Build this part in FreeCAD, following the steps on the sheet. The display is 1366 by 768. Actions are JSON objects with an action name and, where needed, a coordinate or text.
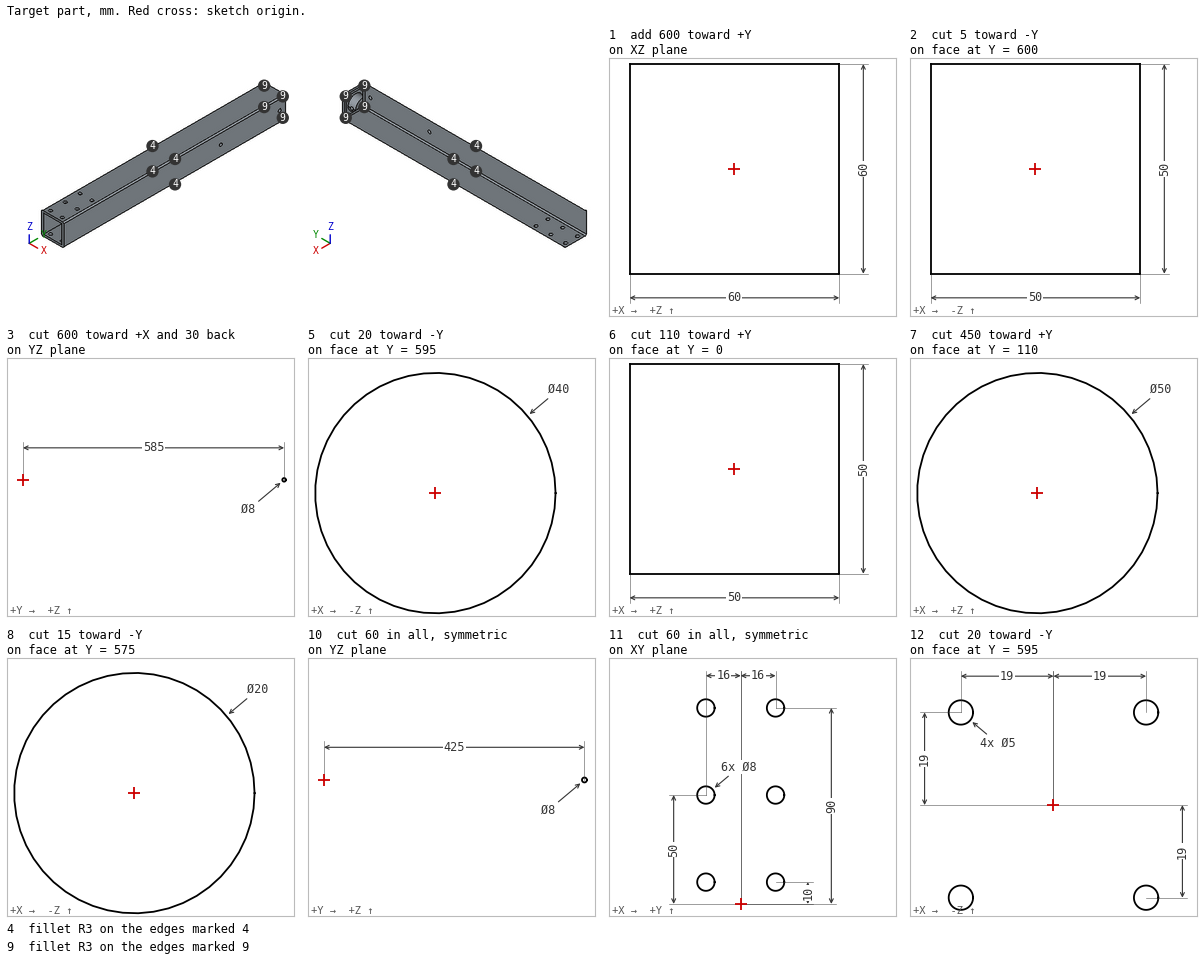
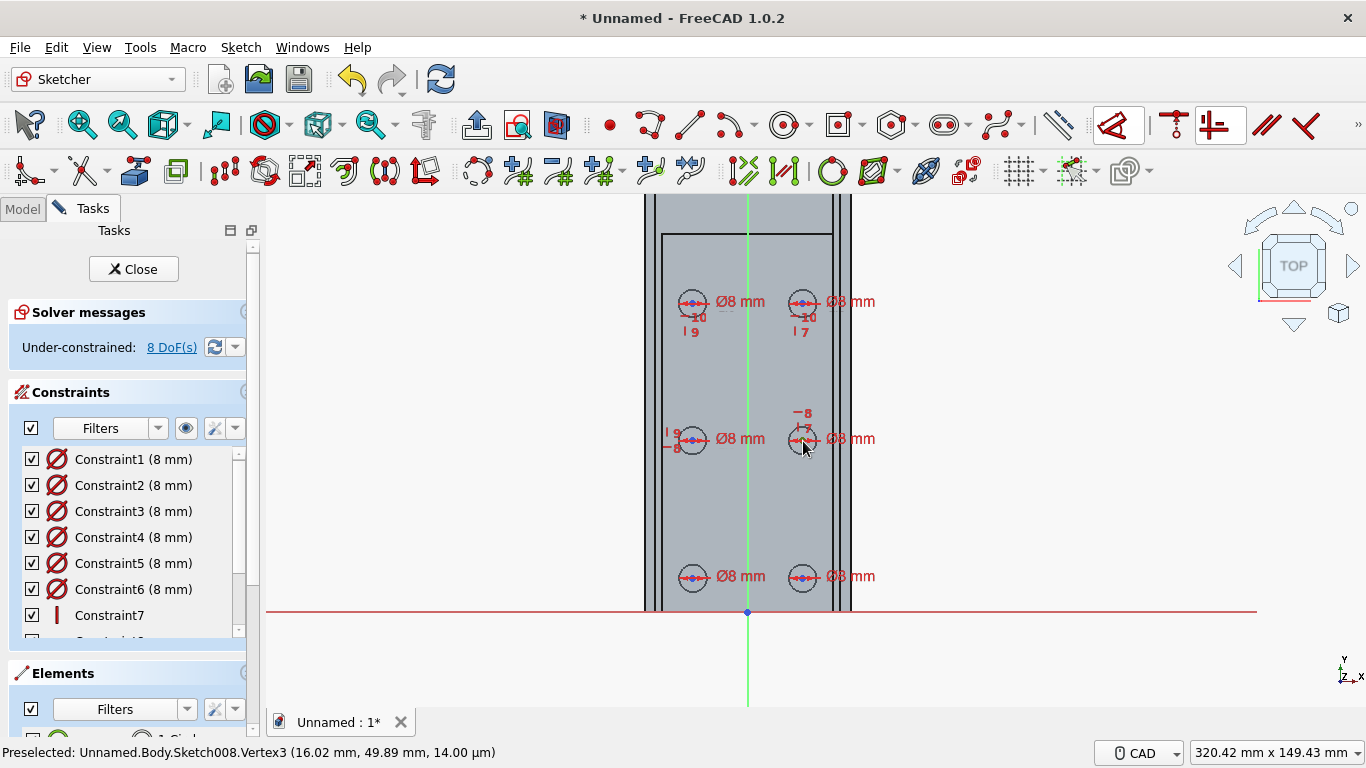
{"action": "left_click", "coordinate": [803, 578]}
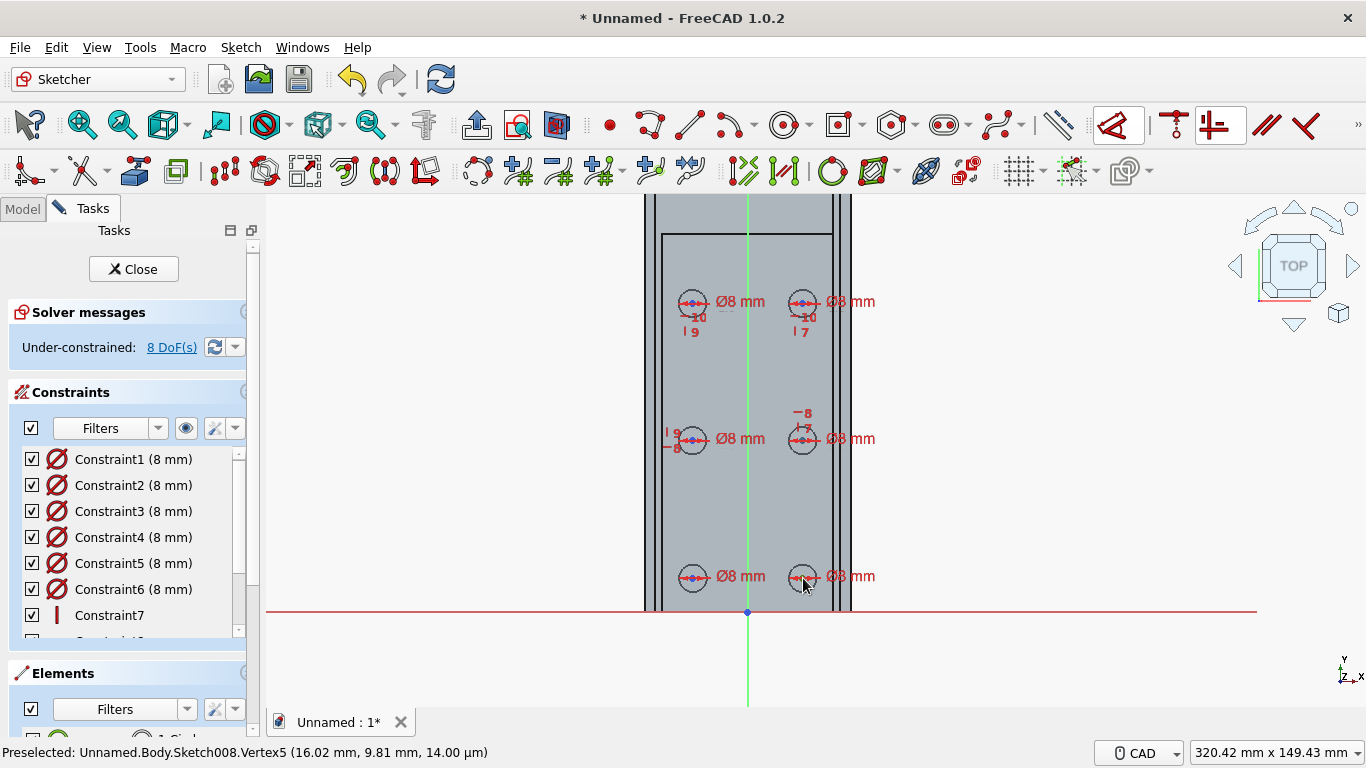
{"action": "key", "text": "v"}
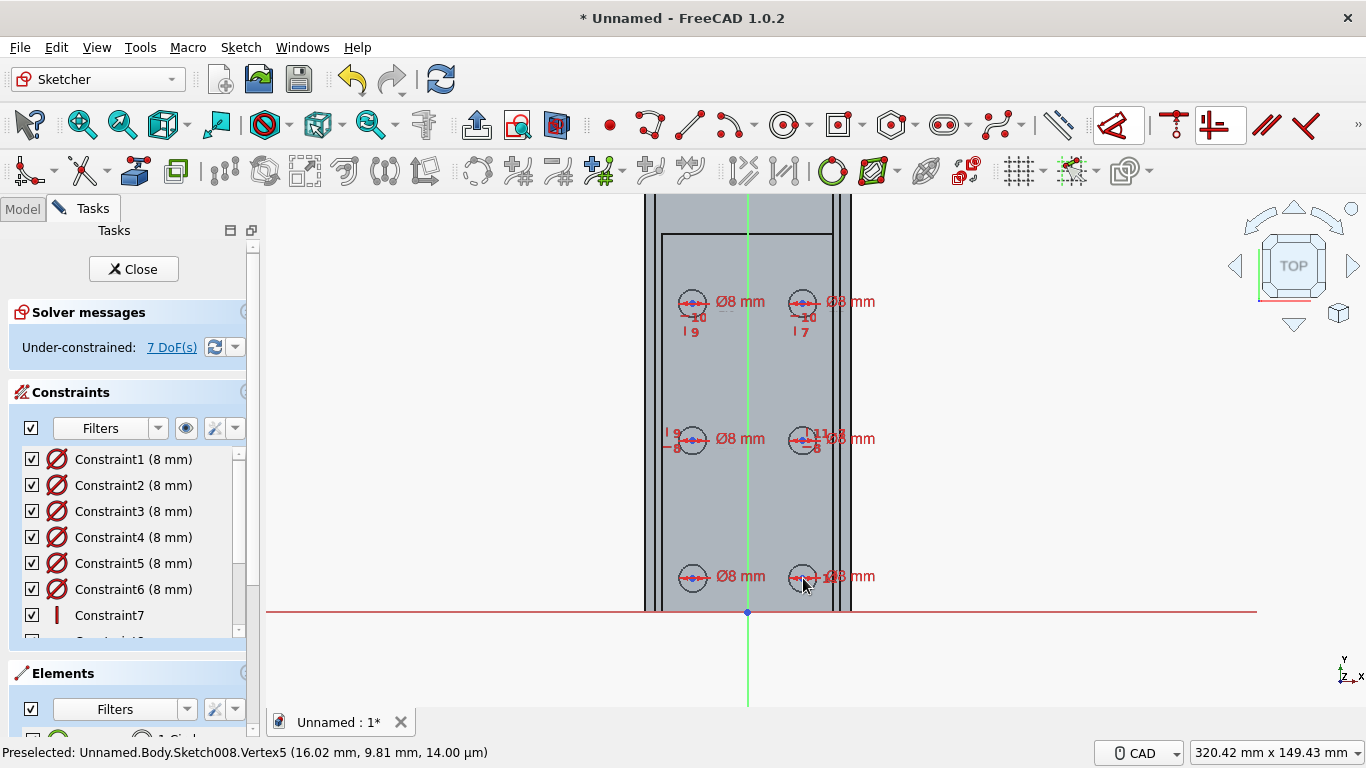
{"action": "left_click", "coordinate": [692, 441]}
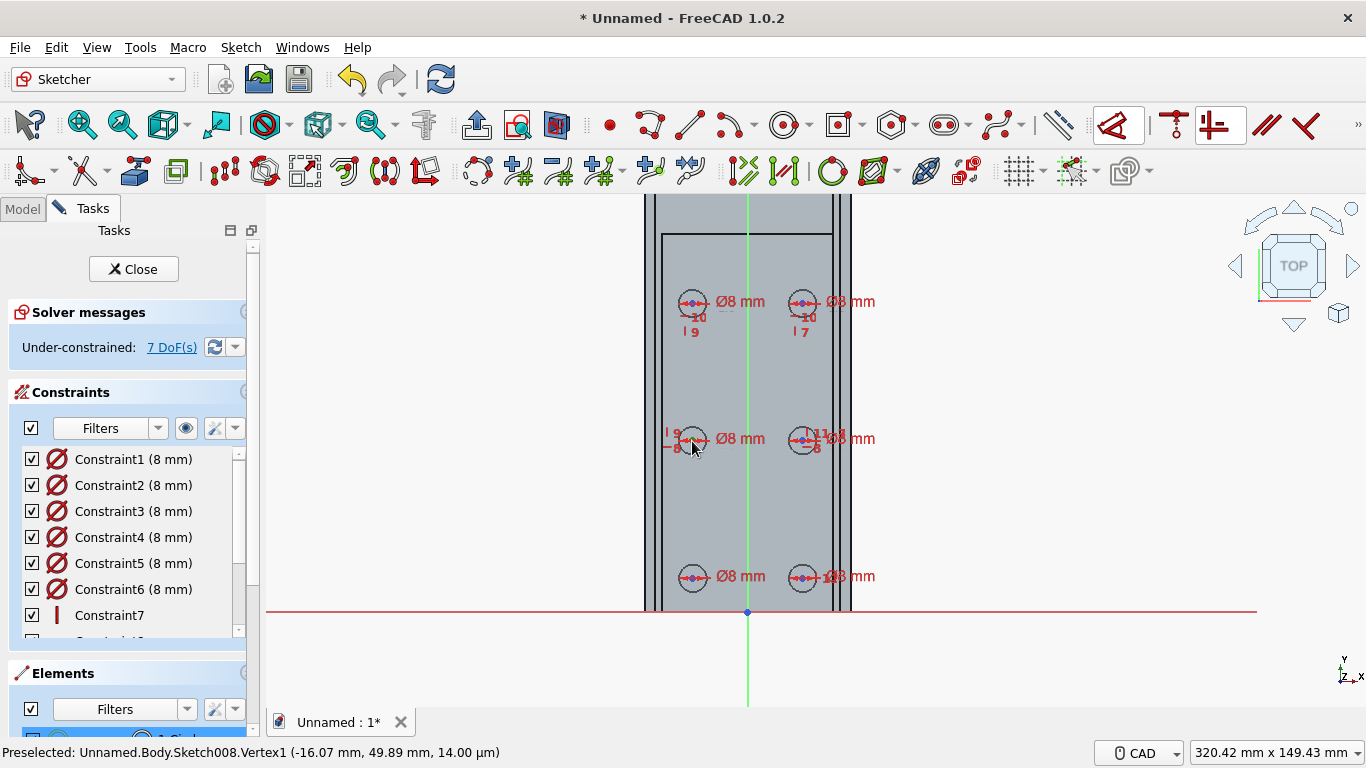
{"action": "left_click", "coordinate": [693, 578]}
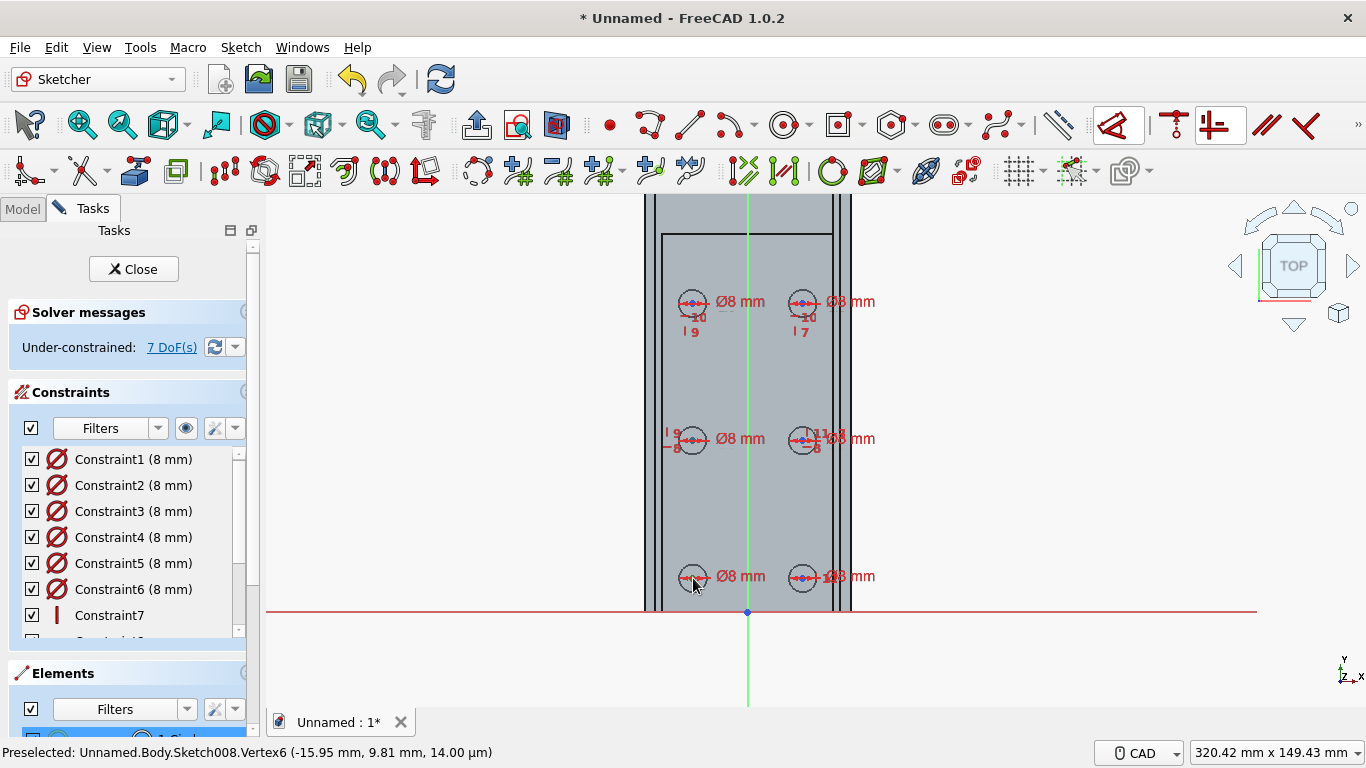
{"action": "left_click", "coordinate": [1240, 126]}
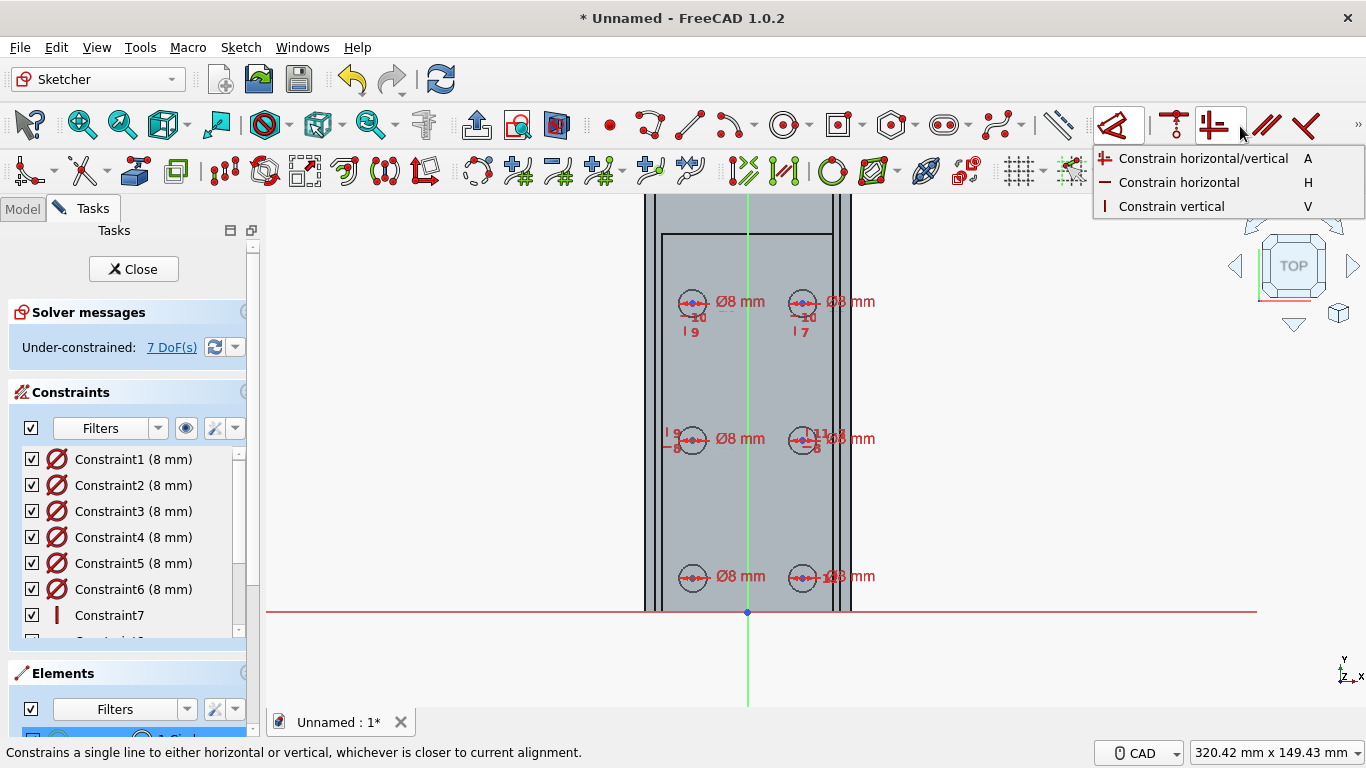
{"action": "left_click", "coordinate": [1229, 206]}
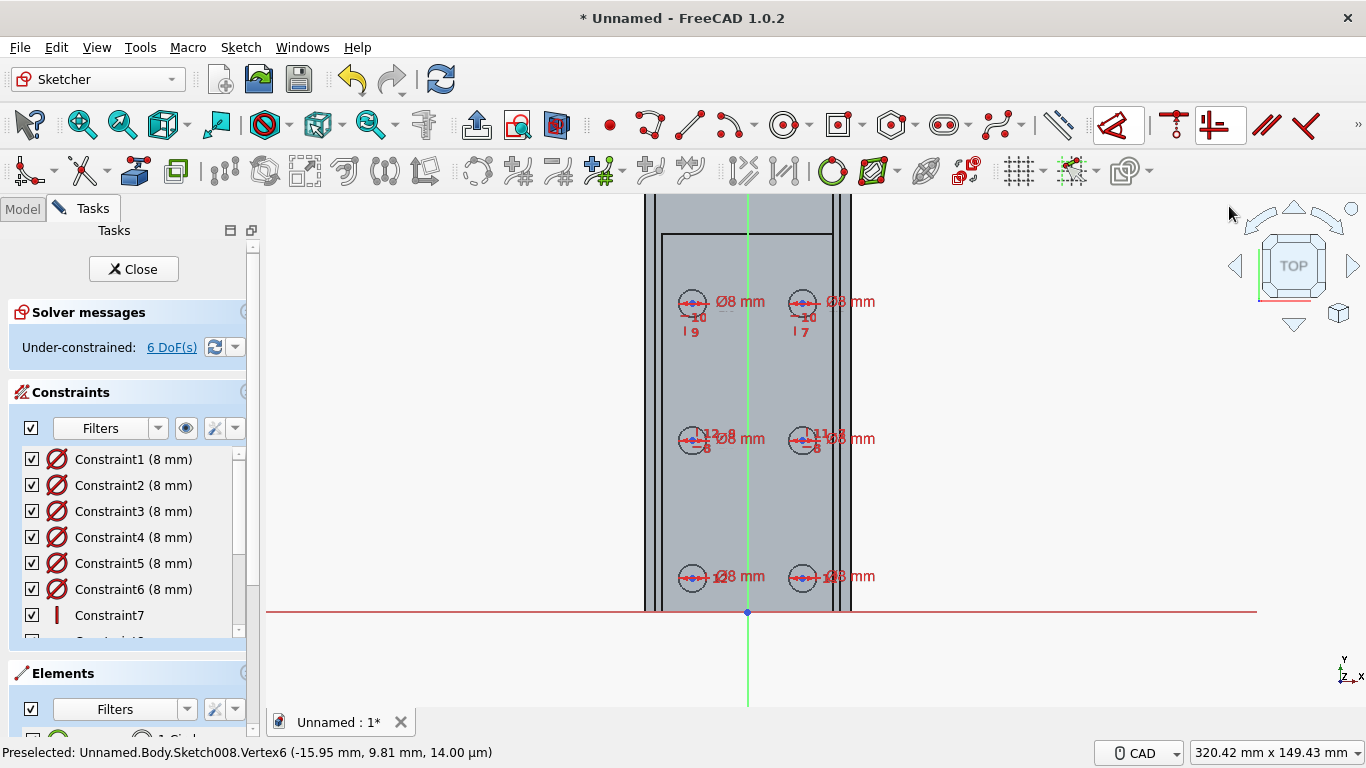
{"action": "left_click", "coordinate": [803, 578]}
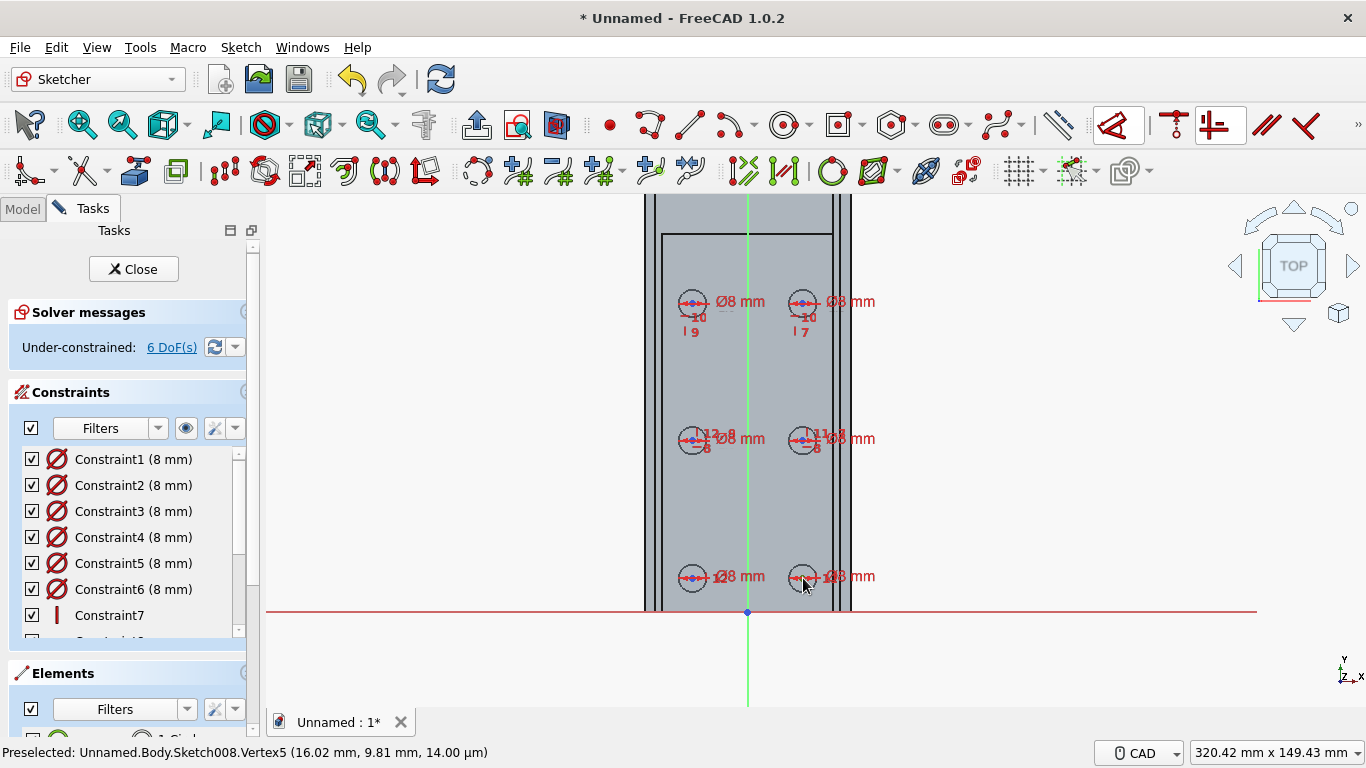
{"action": "left_click", "coordinate": [692, 578]}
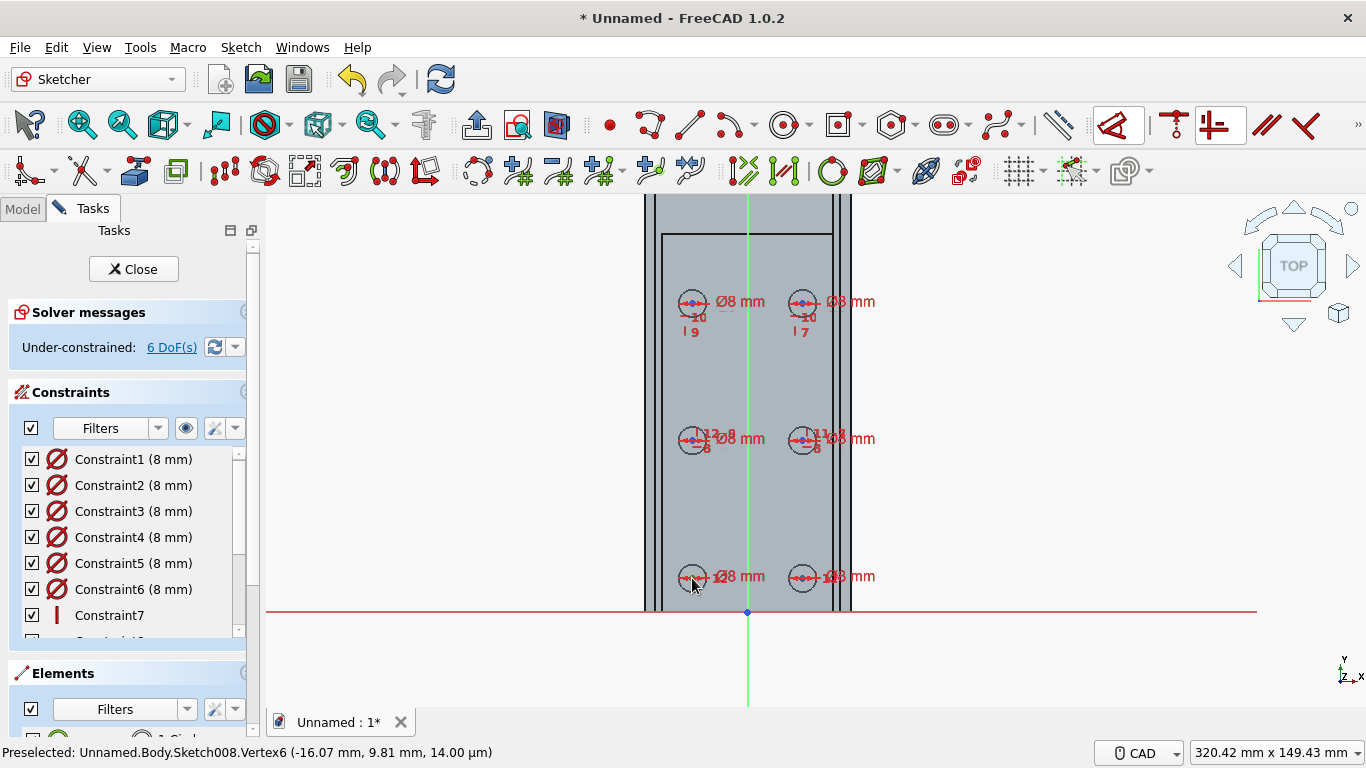
{"action": "left_click", "coordinate": [1240, 126]}